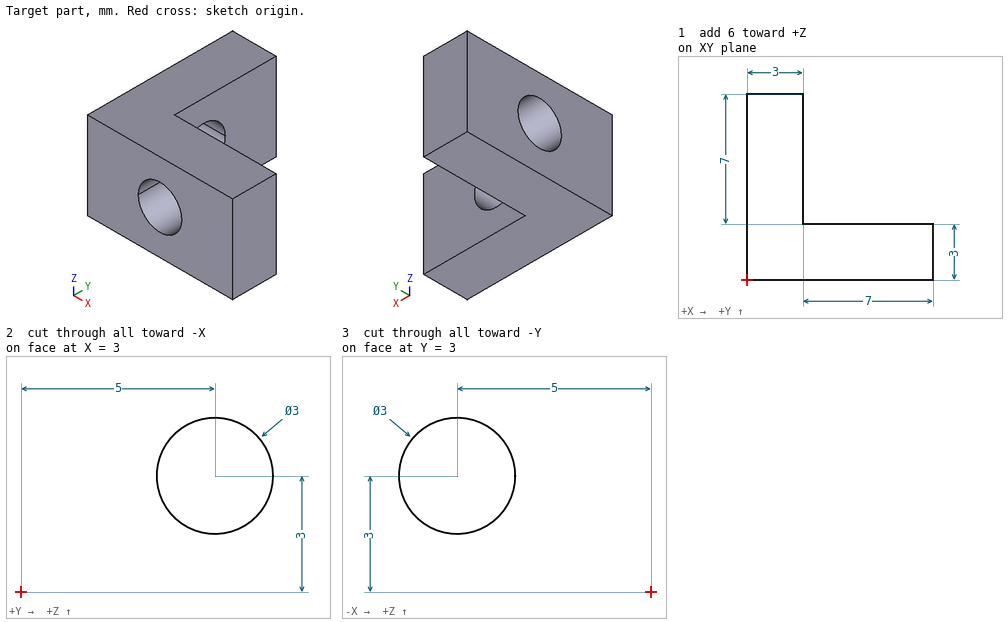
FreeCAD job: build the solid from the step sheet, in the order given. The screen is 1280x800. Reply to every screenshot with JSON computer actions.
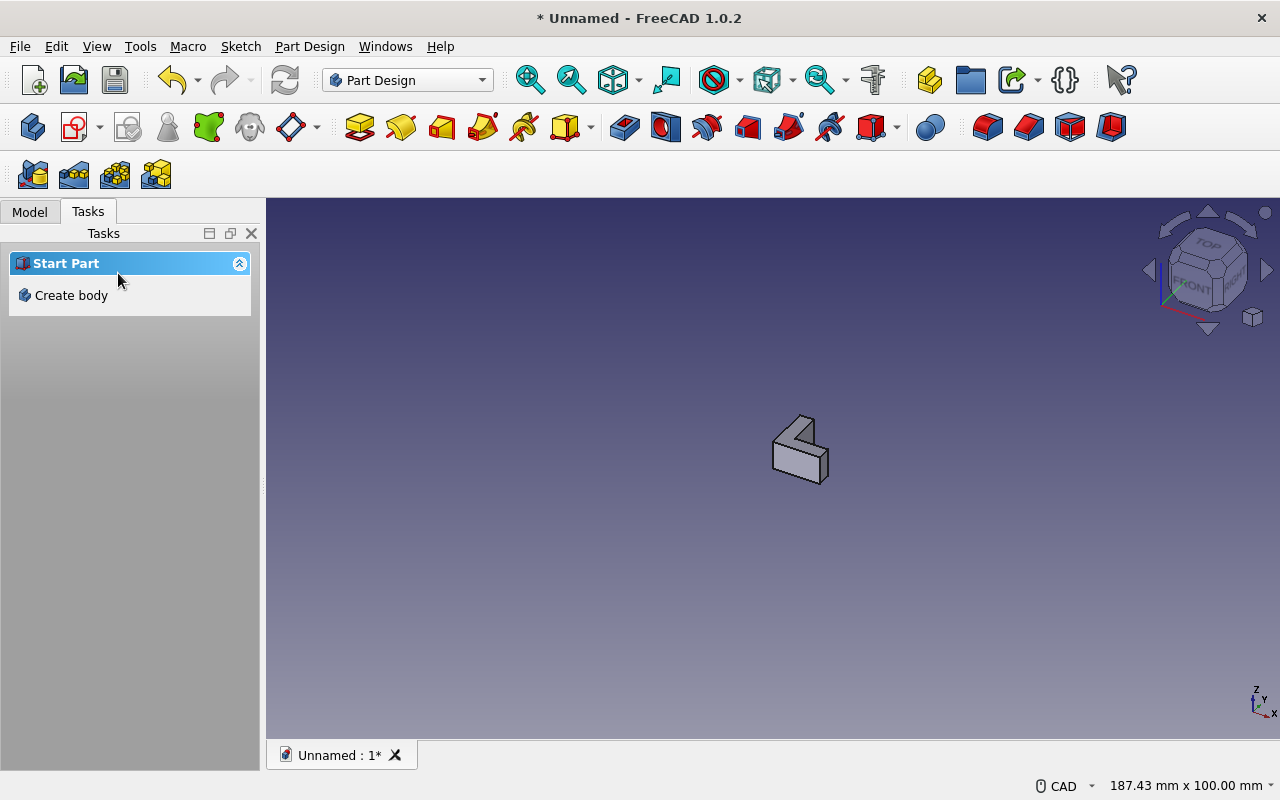
{"action": "left_click", "coordinate": [531, 80]}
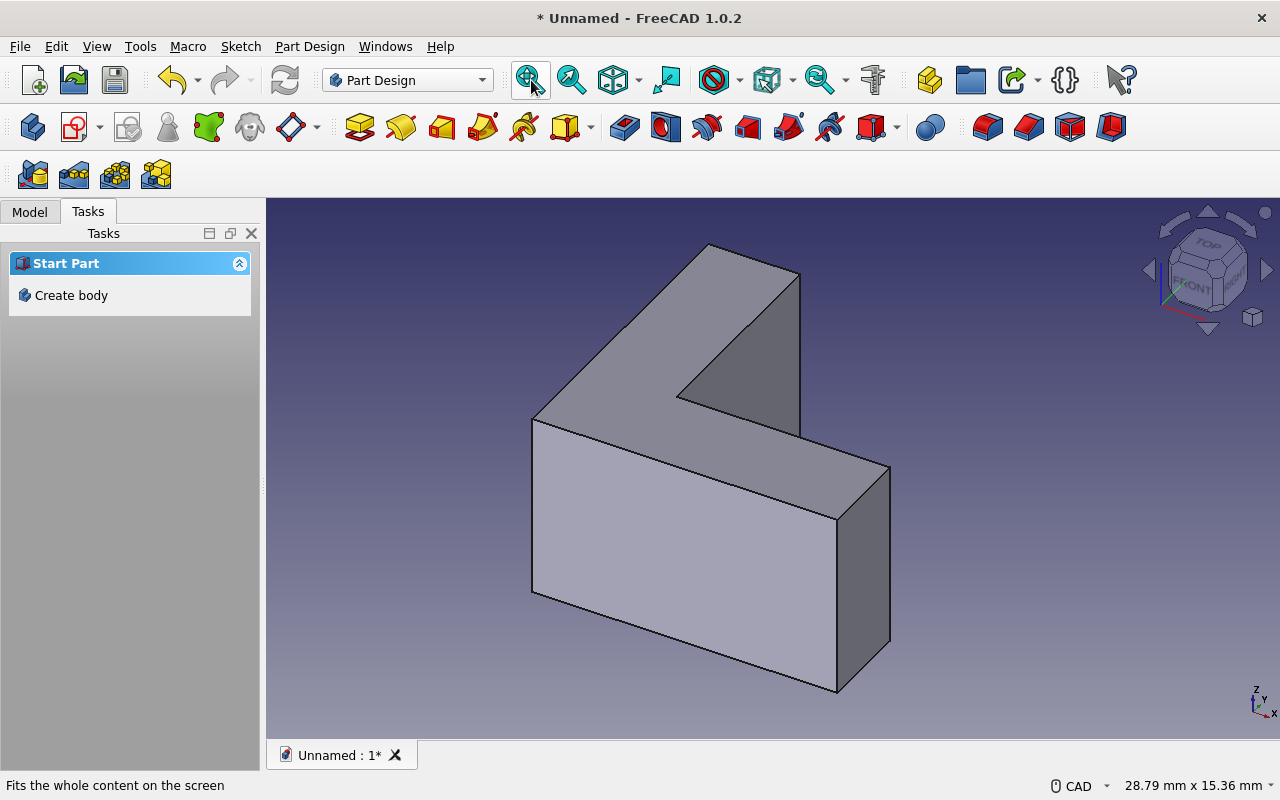
{"action": "left_click", "coordinate": [756, 404]}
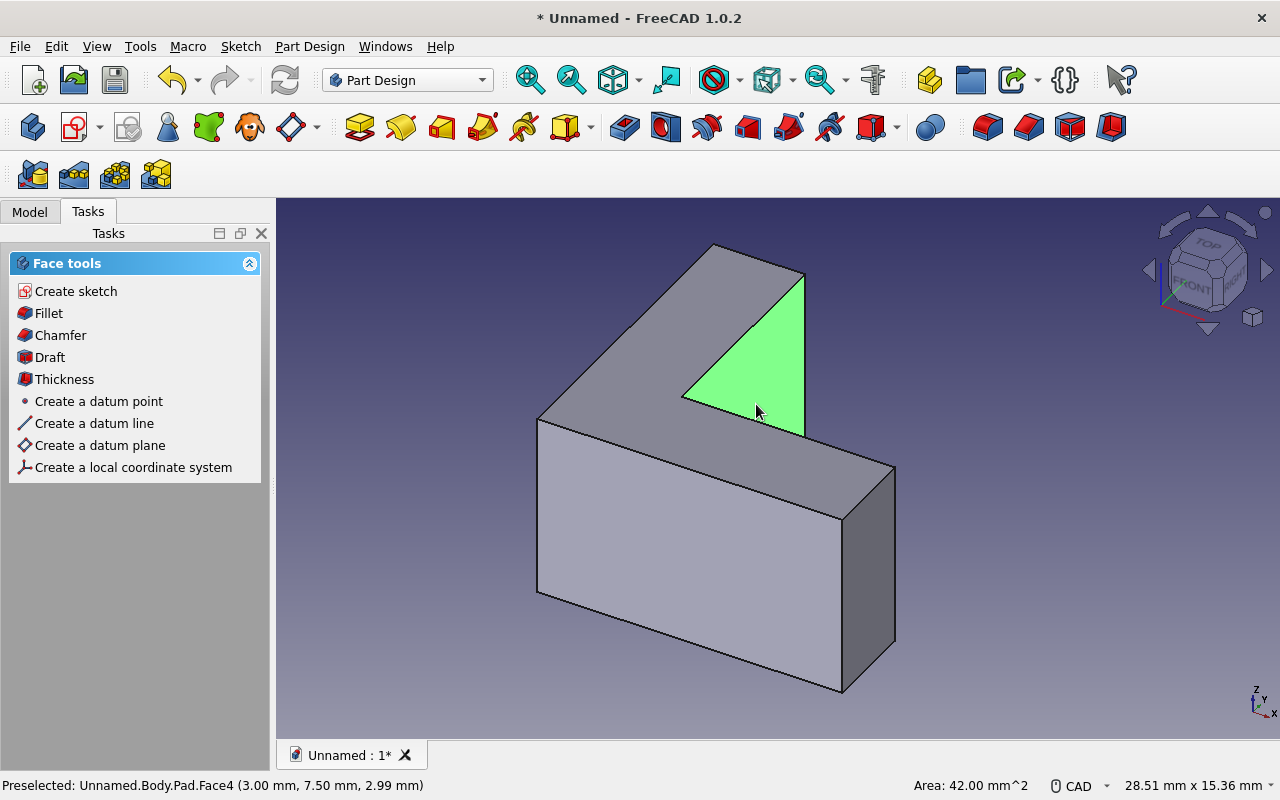
{"action": "left_click", "coordinate": [74, 128]}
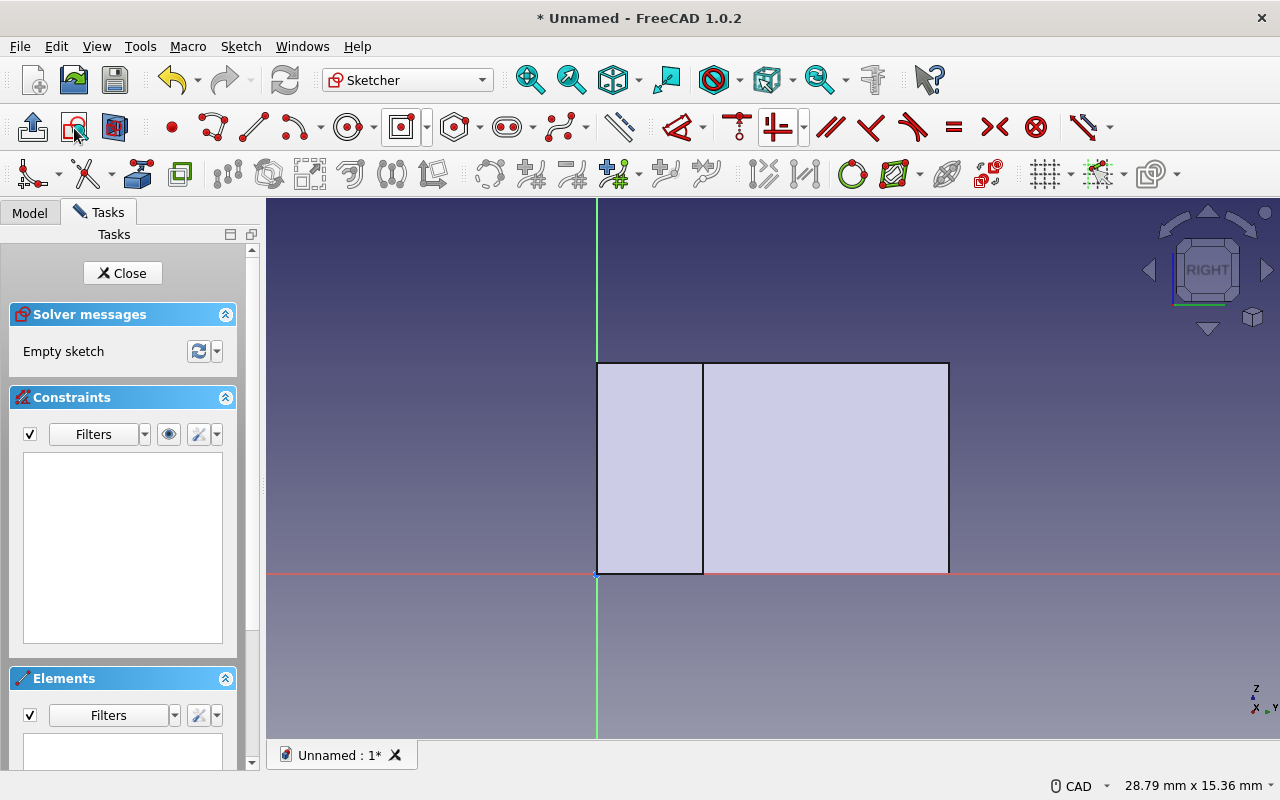
{"action": "left_click", "coordinate": [115, 128]}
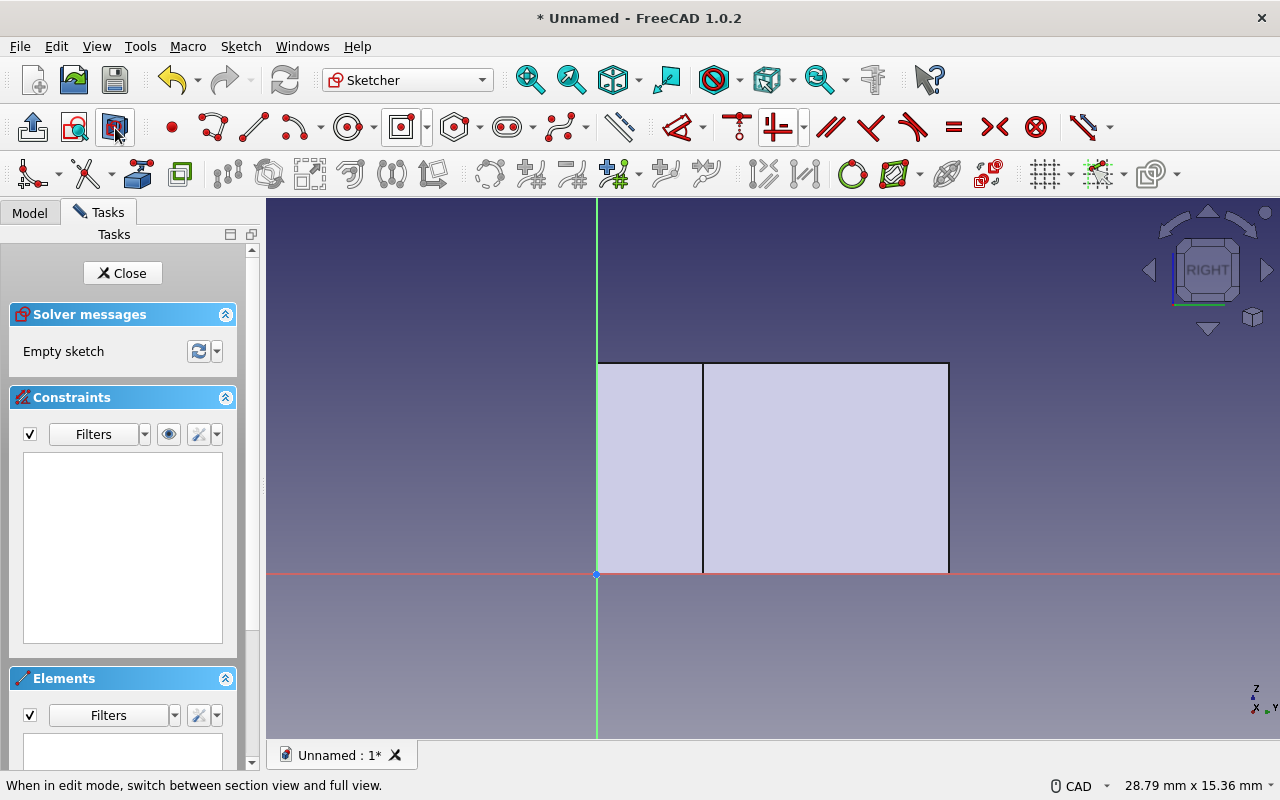
{"action": "scroll", "coordinate": [717, 516], "scroll_direction": "up", "scroll_amount": 4}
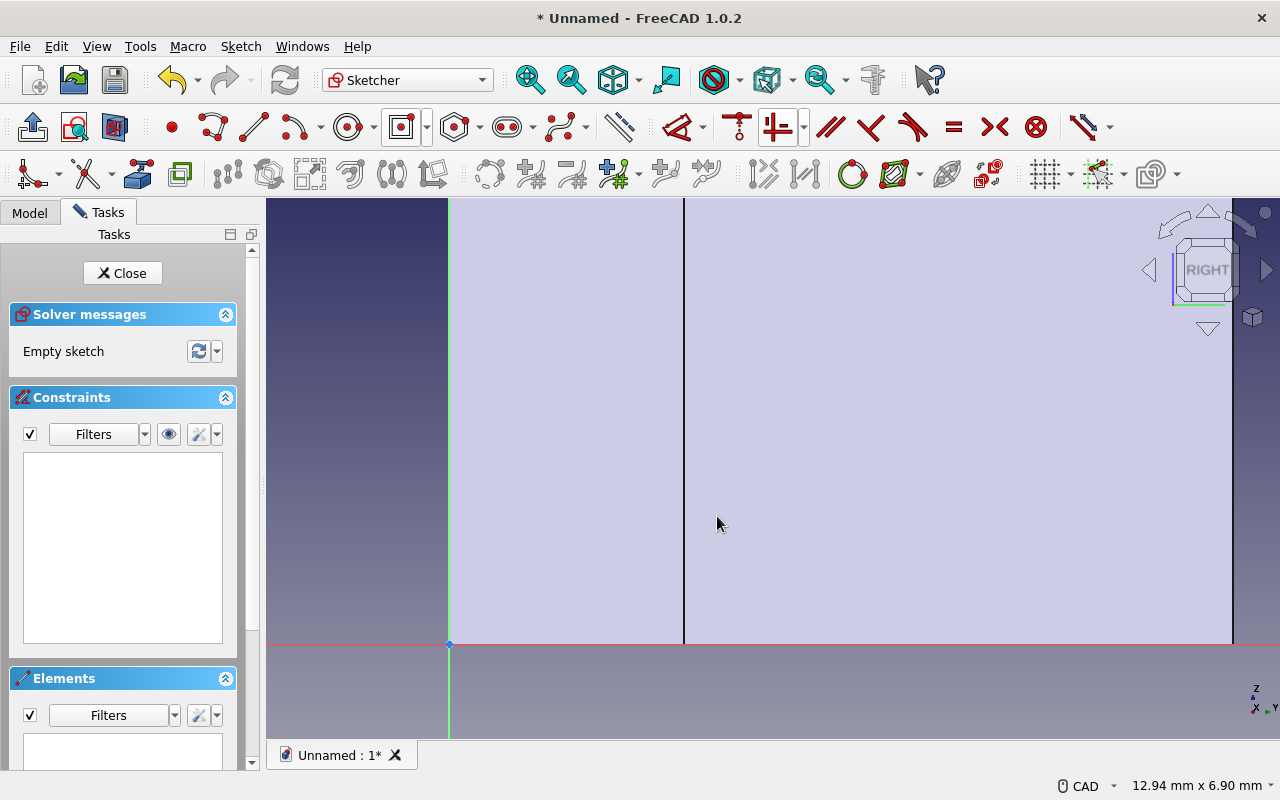
{"action": "left_click", "coordinate": [348, 128]}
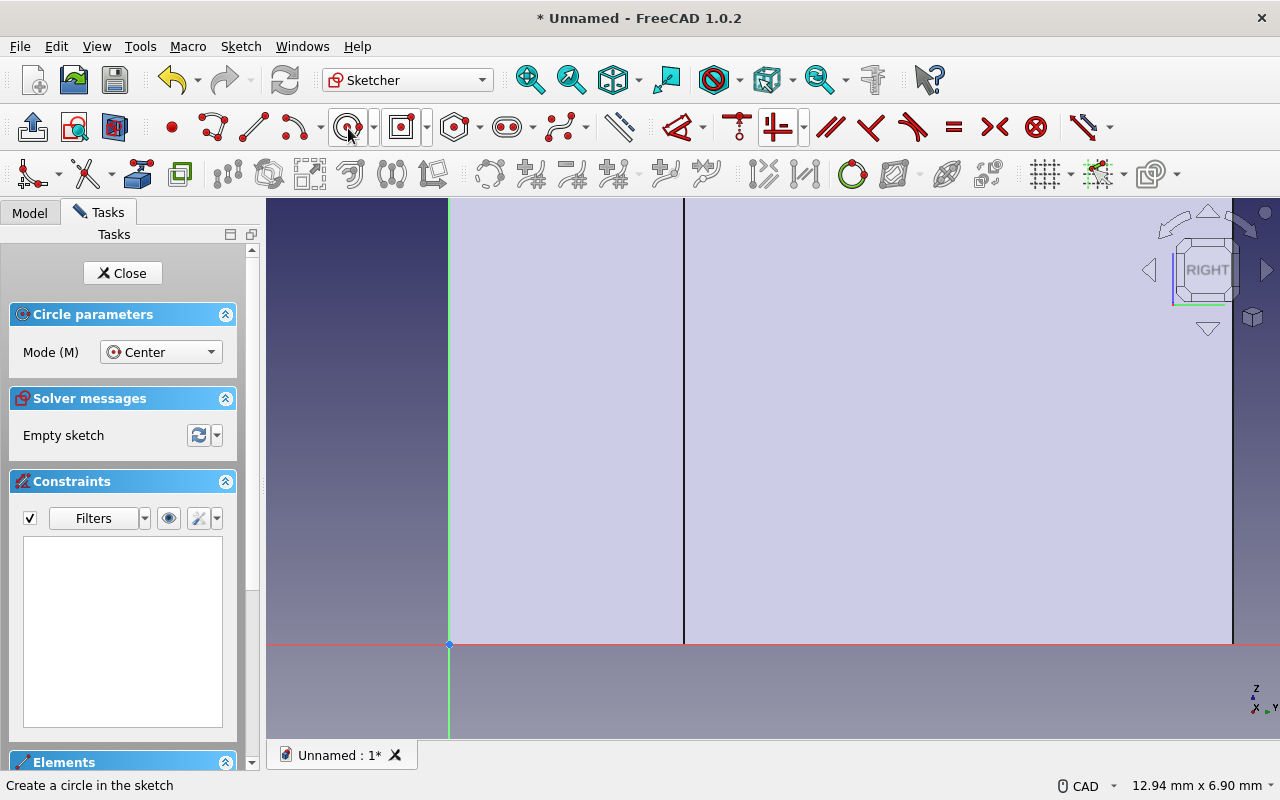
{"action": "left_click", "coordinate": [841, 410]}
{"action": "left_click", "coordinate": [924, 326]}
{"action": "key", "text": "Escape"}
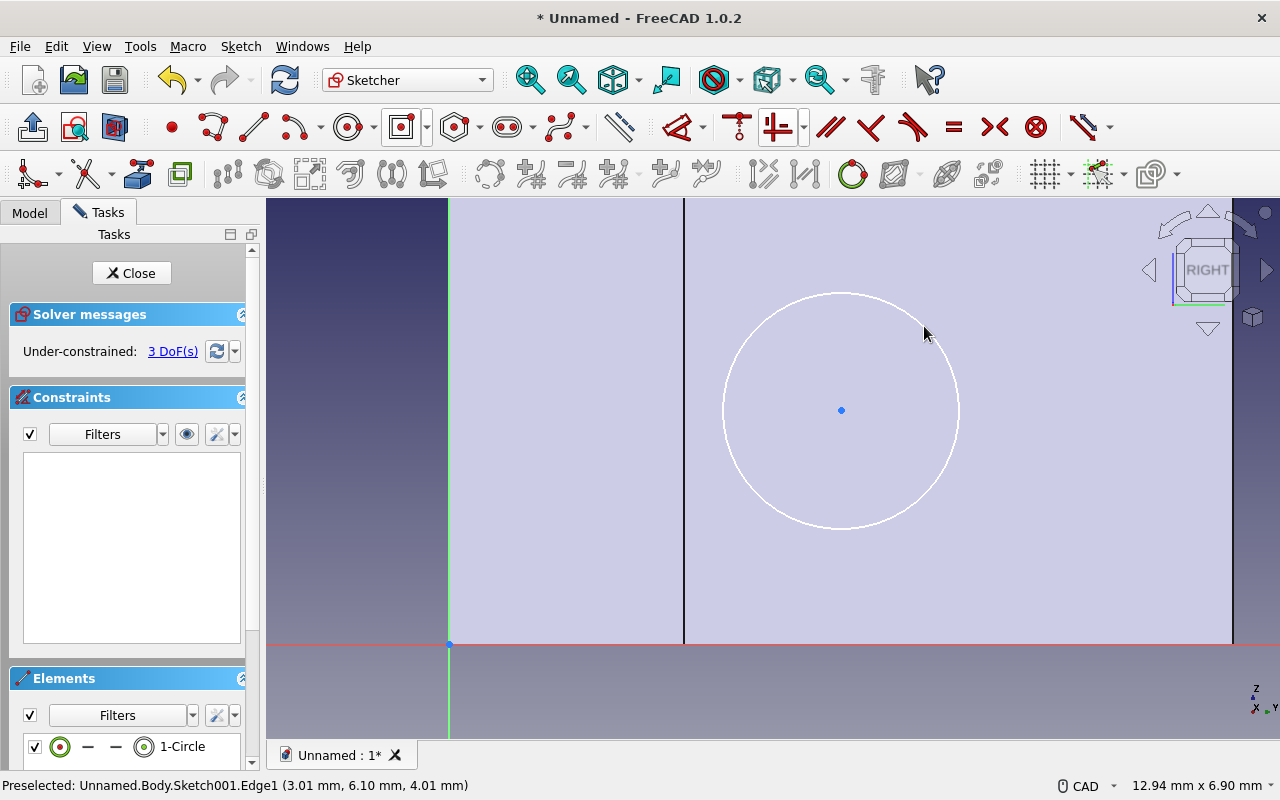
{"action": "left_click", "coordinate": [676, 128]}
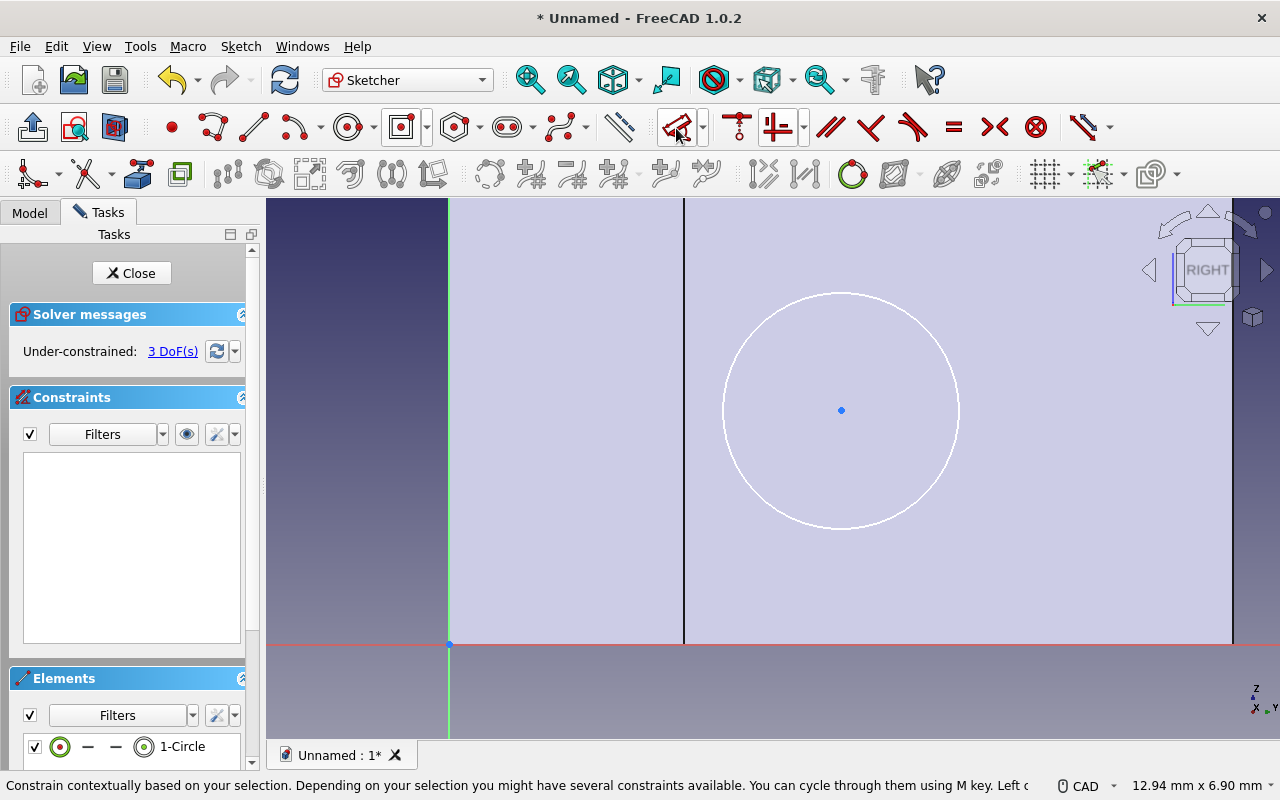
{"action": "left_click", "coordinate": [924, 327]}
{"action": "left_click", "coordinate": [946, 304]}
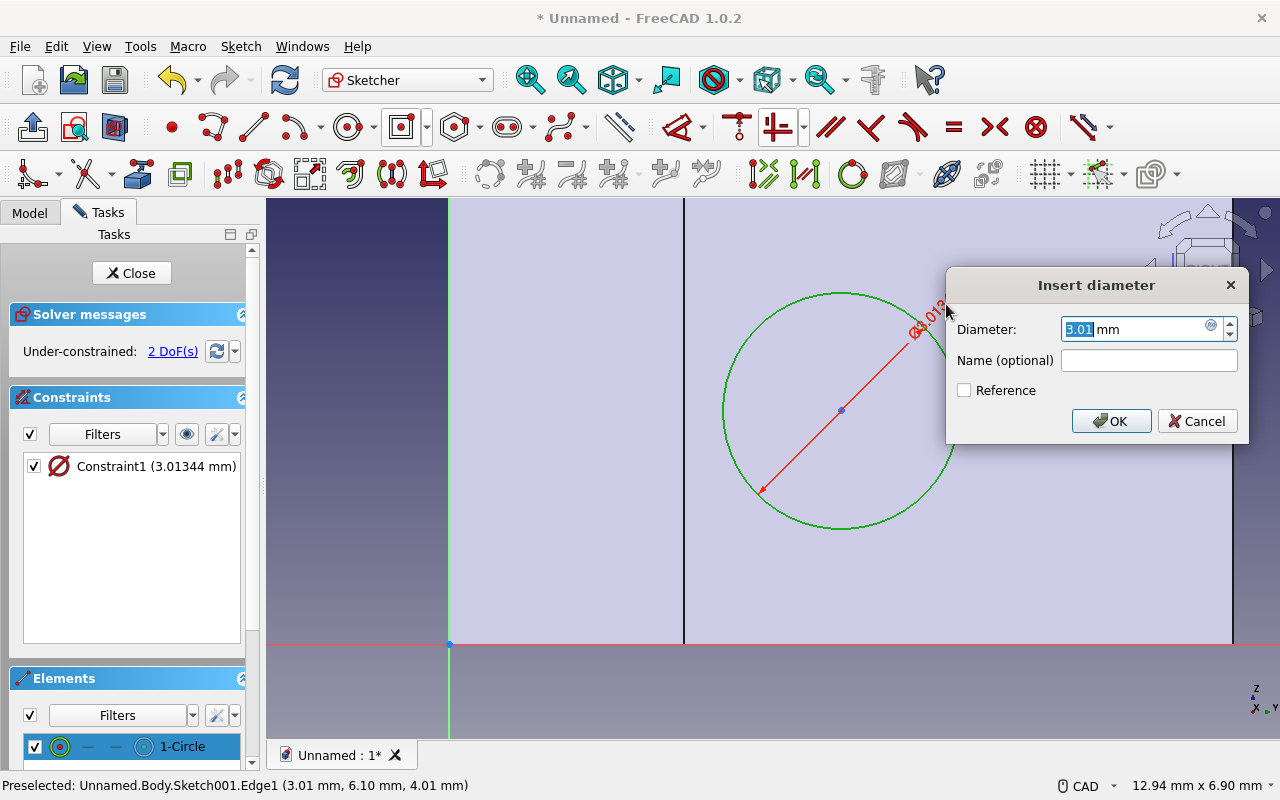
{"action": "type", "text": "3"}
{"action": "key", "text": "Return"}